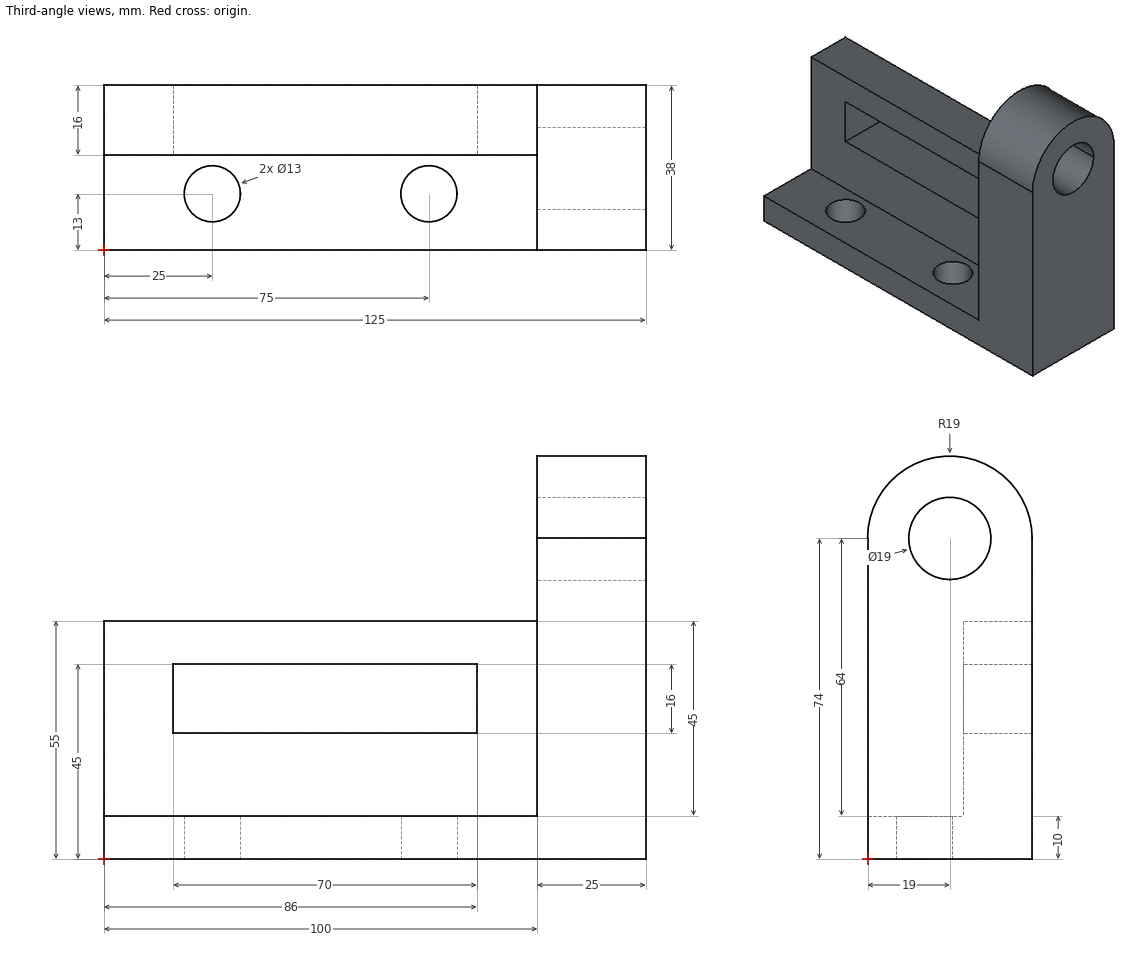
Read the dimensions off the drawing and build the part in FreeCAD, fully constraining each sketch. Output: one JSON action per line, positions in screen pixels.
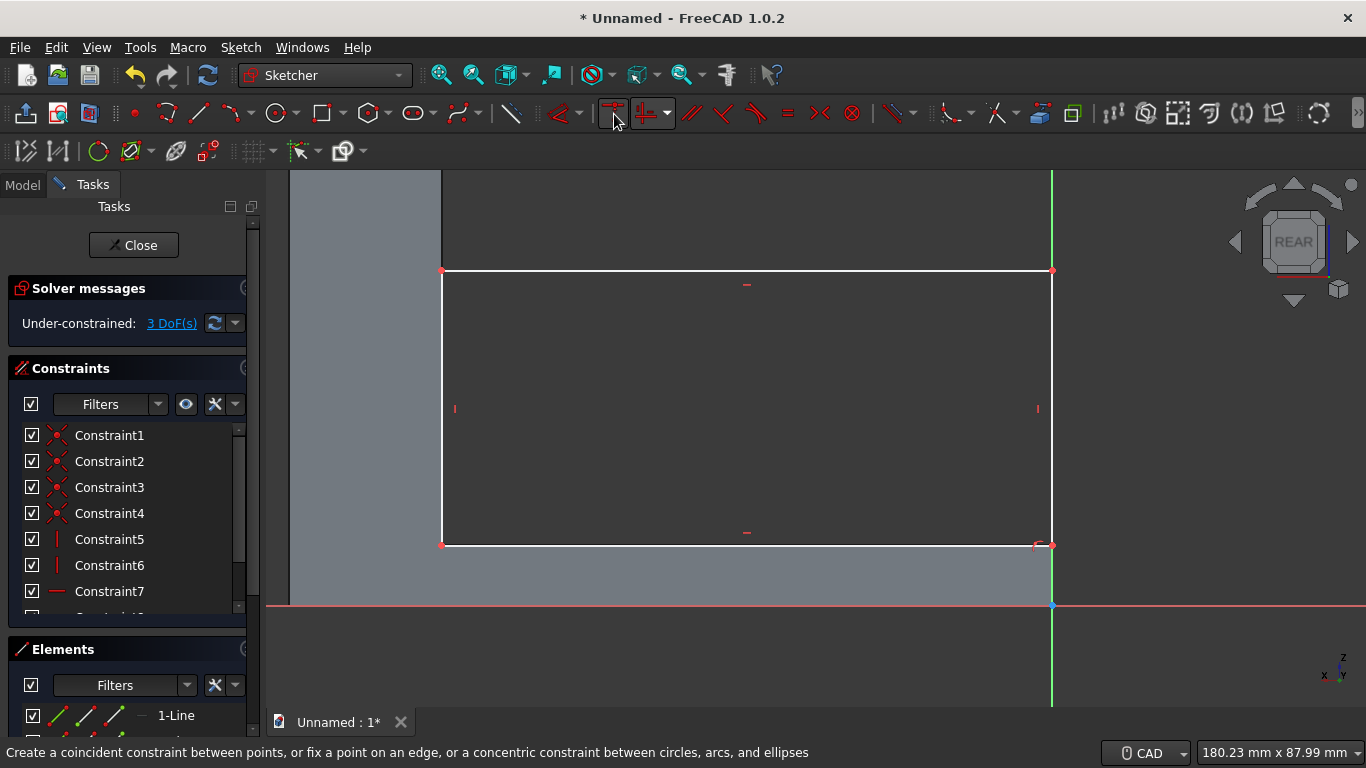
{"action": "left_click", "coordinate": [558, 114]}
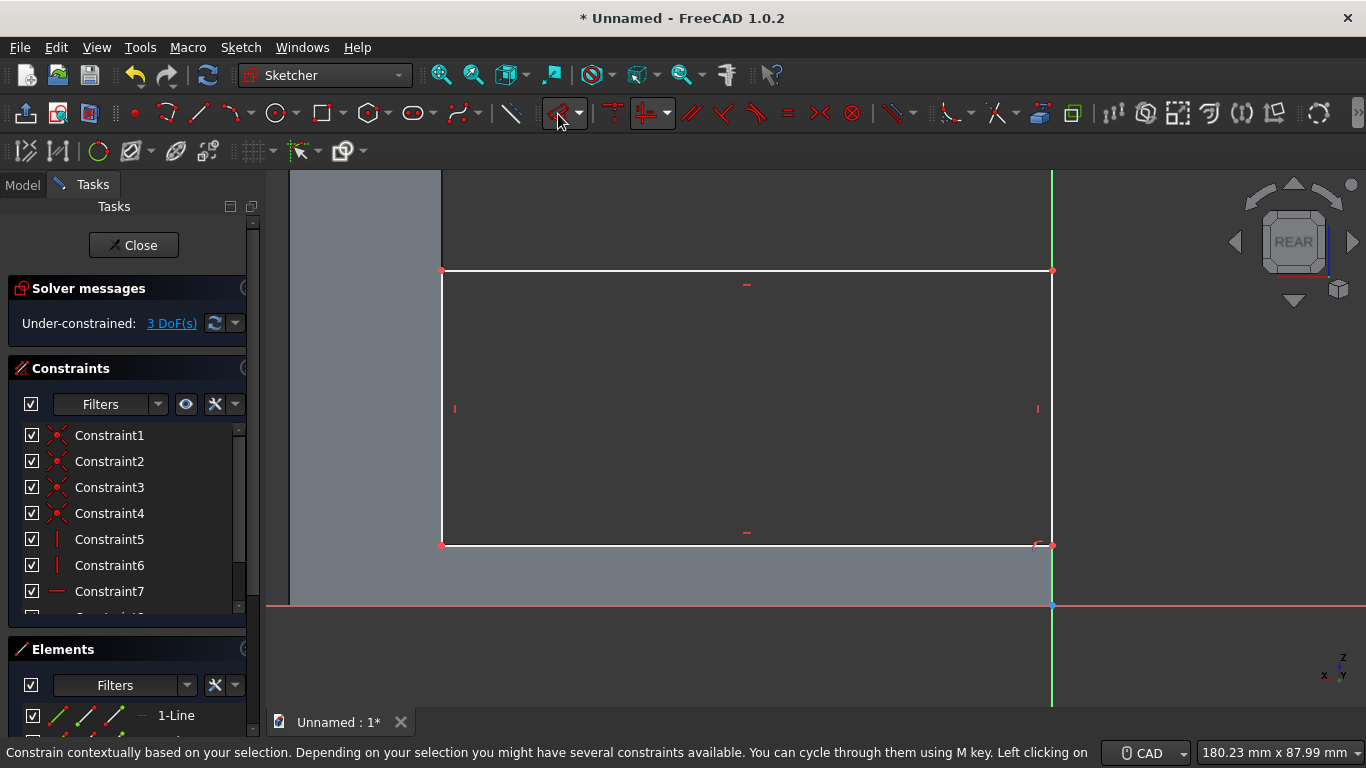
{"action": "left_click", "coordinate": [442, 353]}
{"action": "left_click", "coordinate": [408, 408]}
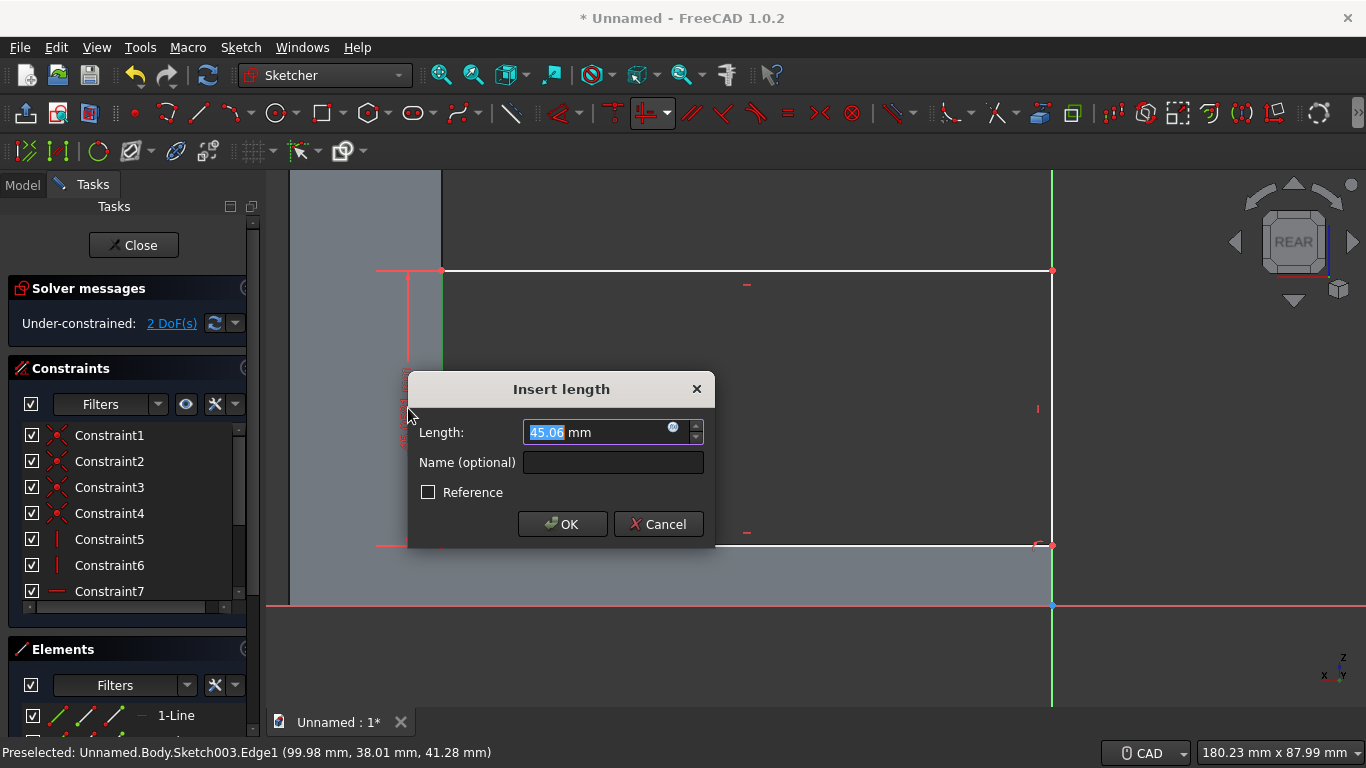
{"action": "type", "text": "45"}
{"action": "key", "text": "Return"}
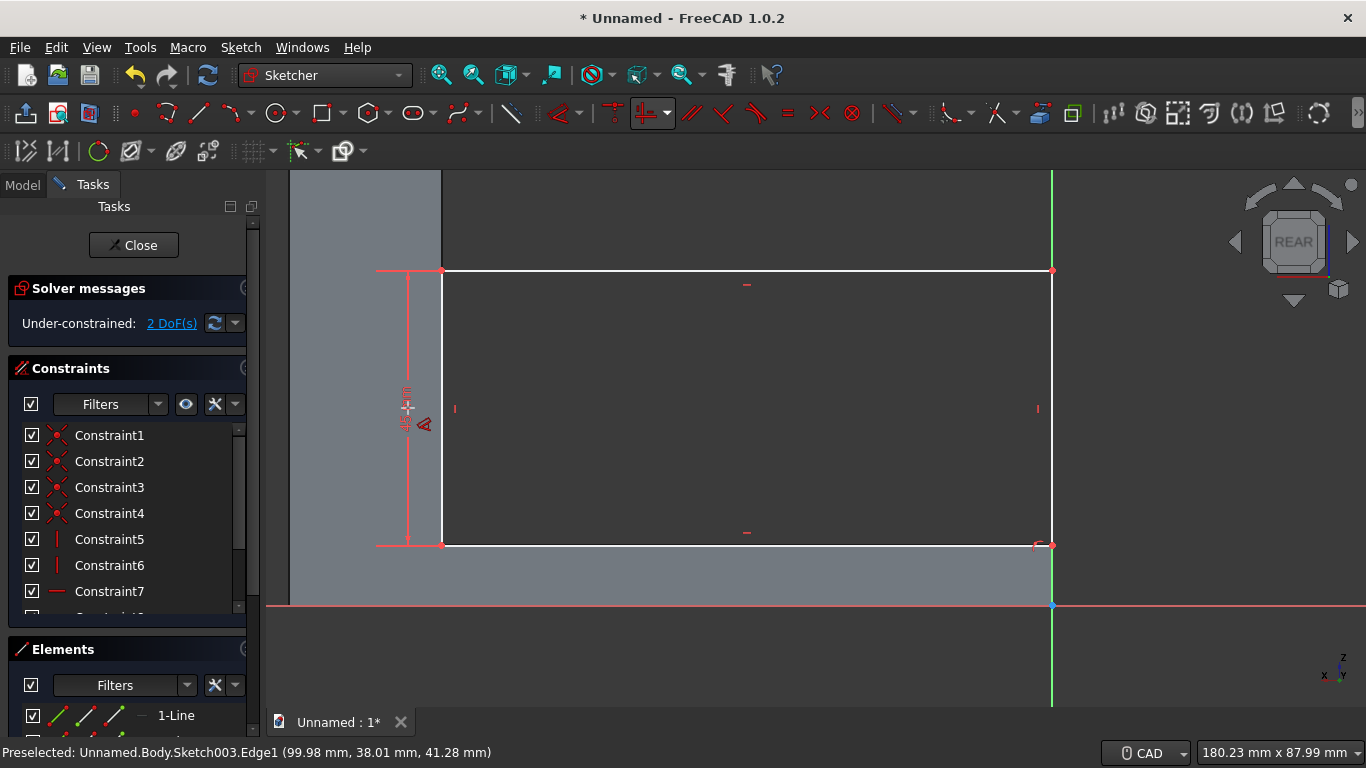
{"action": "left_click", "coordinate": [625, 546]}
{"action": "left_click", "coordinate": [747, 580]}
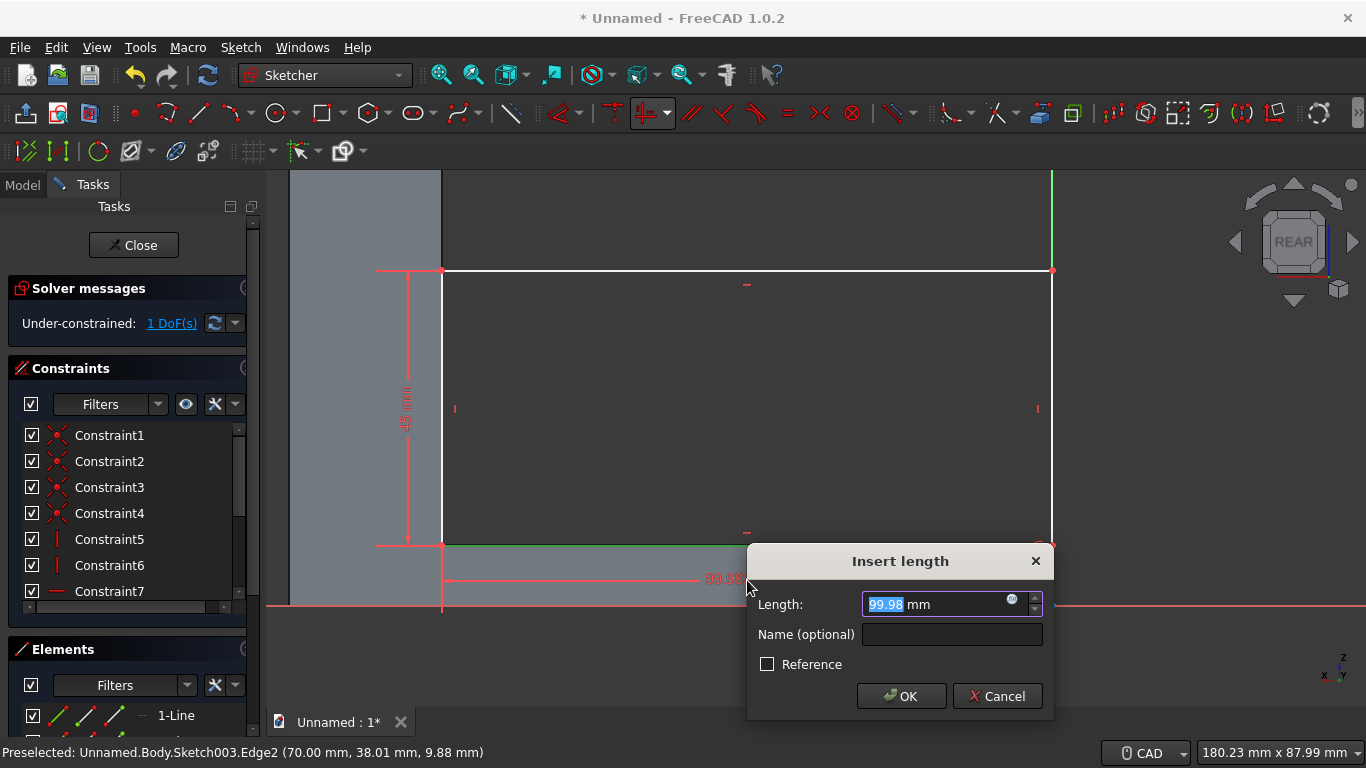
{"action": "type", "text": "100"}
{"action": "key", "text": "Return"}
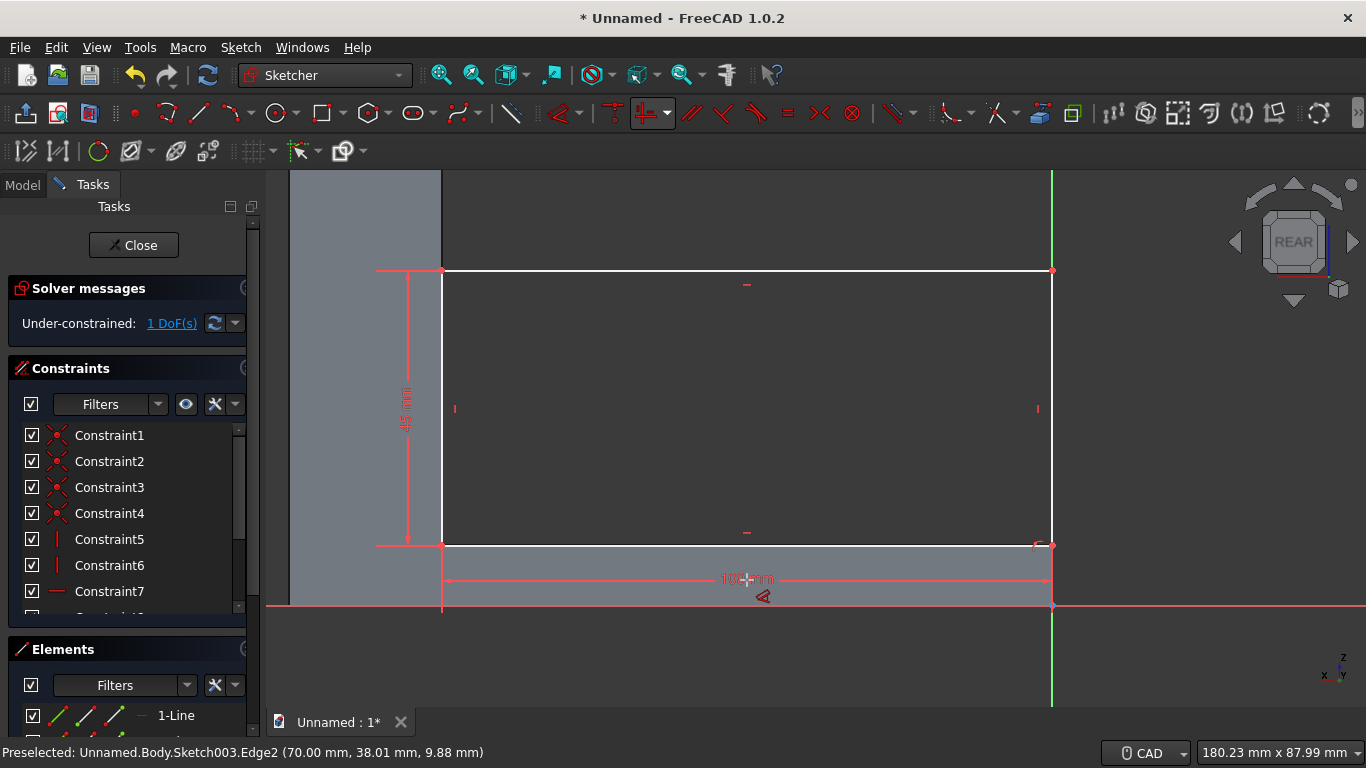
{"action": "left_click", "coordinate": [442, 271]}
{"action": "left_click", "coordinate": [1086, 438]}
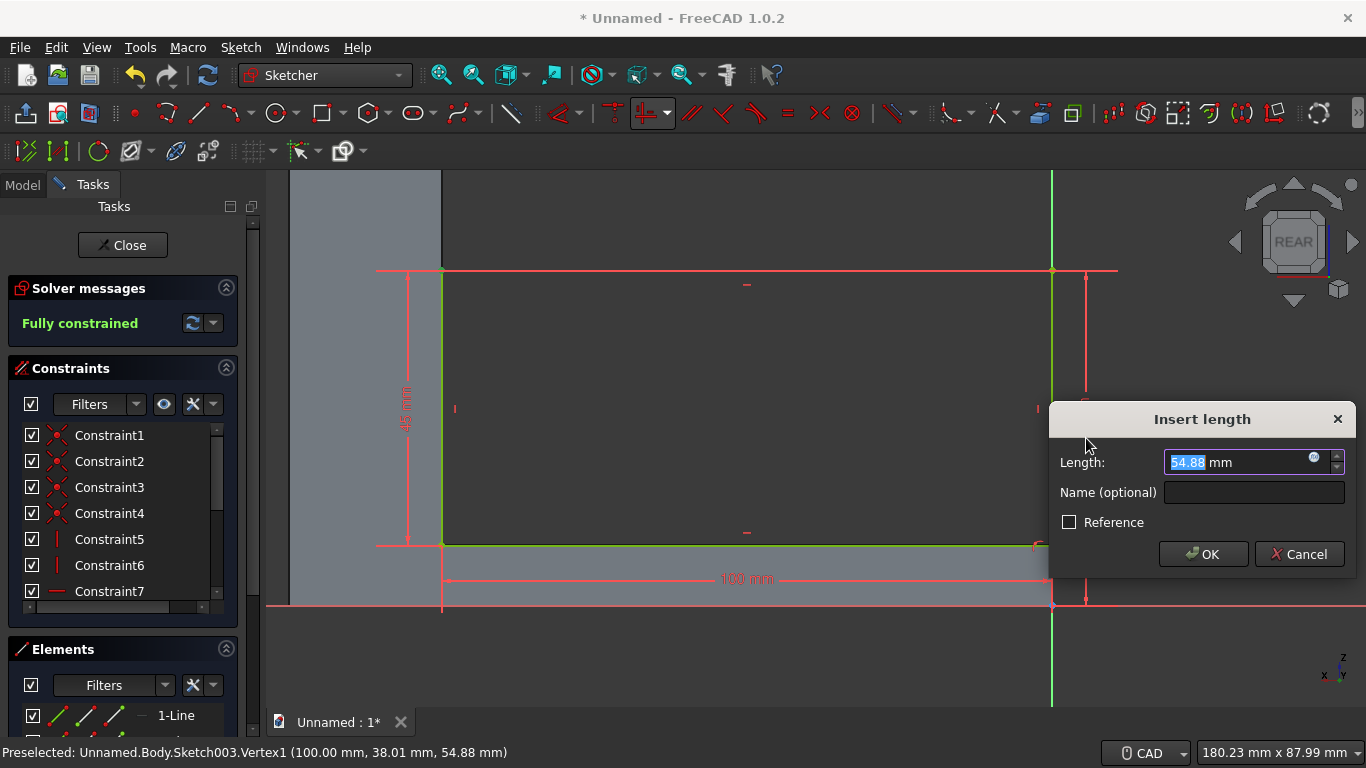
{"action": "type", "text": "55"}
{"action": "key", "text": "Return"}
{"action": "key", "text": "Escape"}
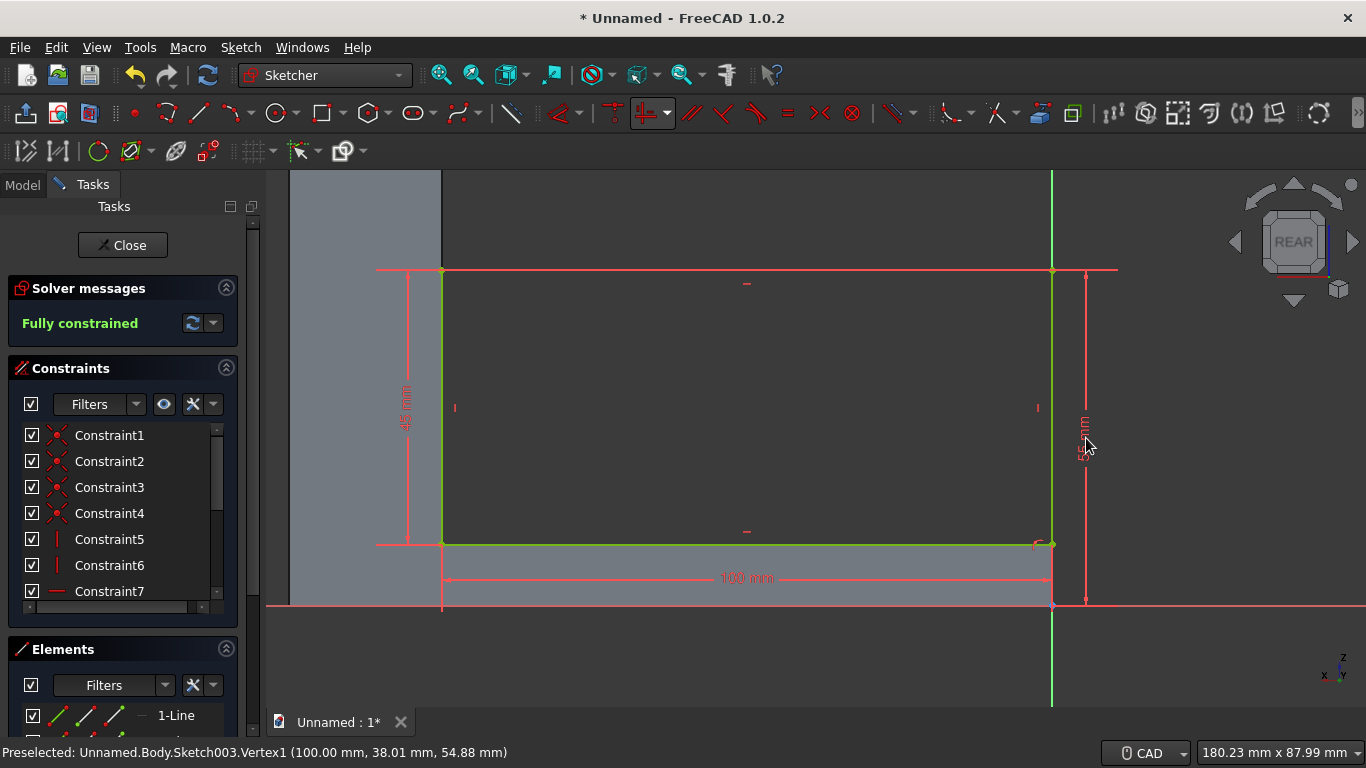
{"action": "left_click", "coordinate": [123, 245]}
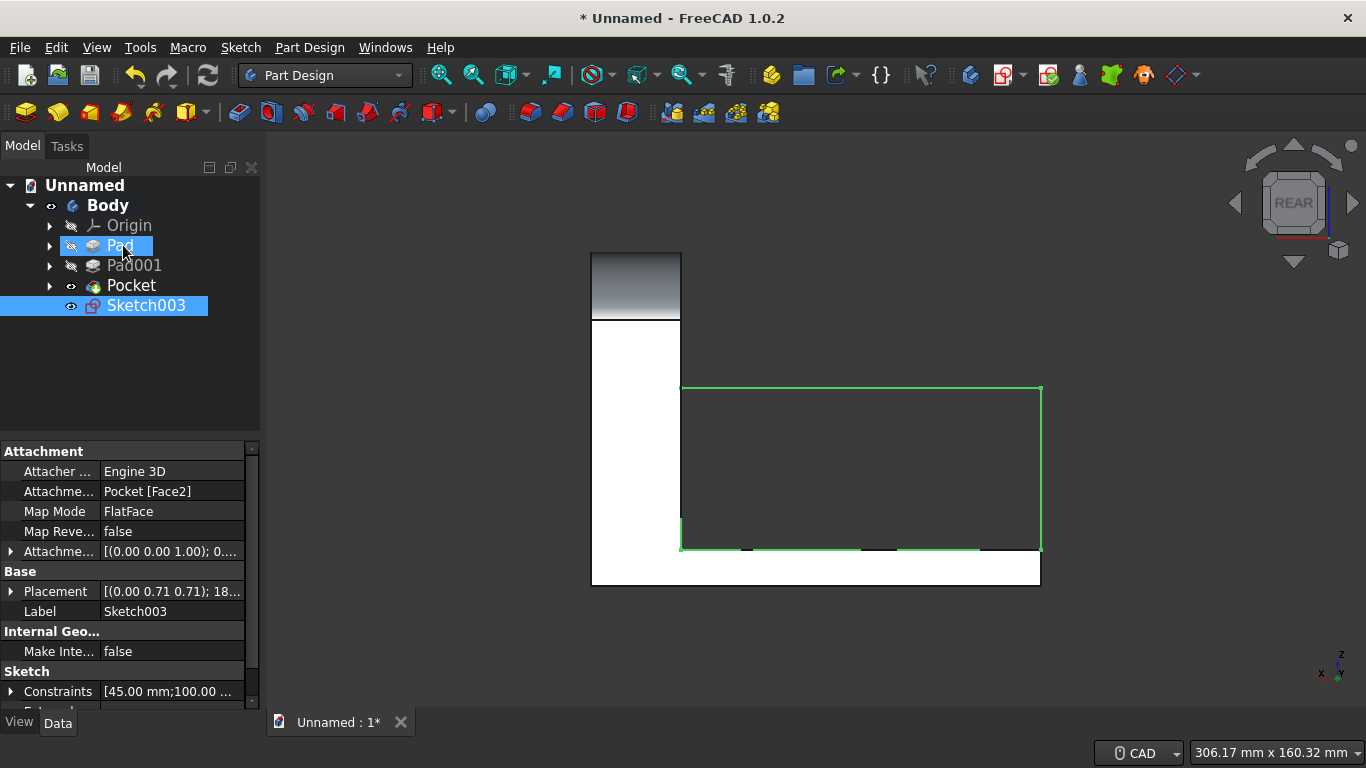
{"action": "left_click", "coordinate": [26, 112]}